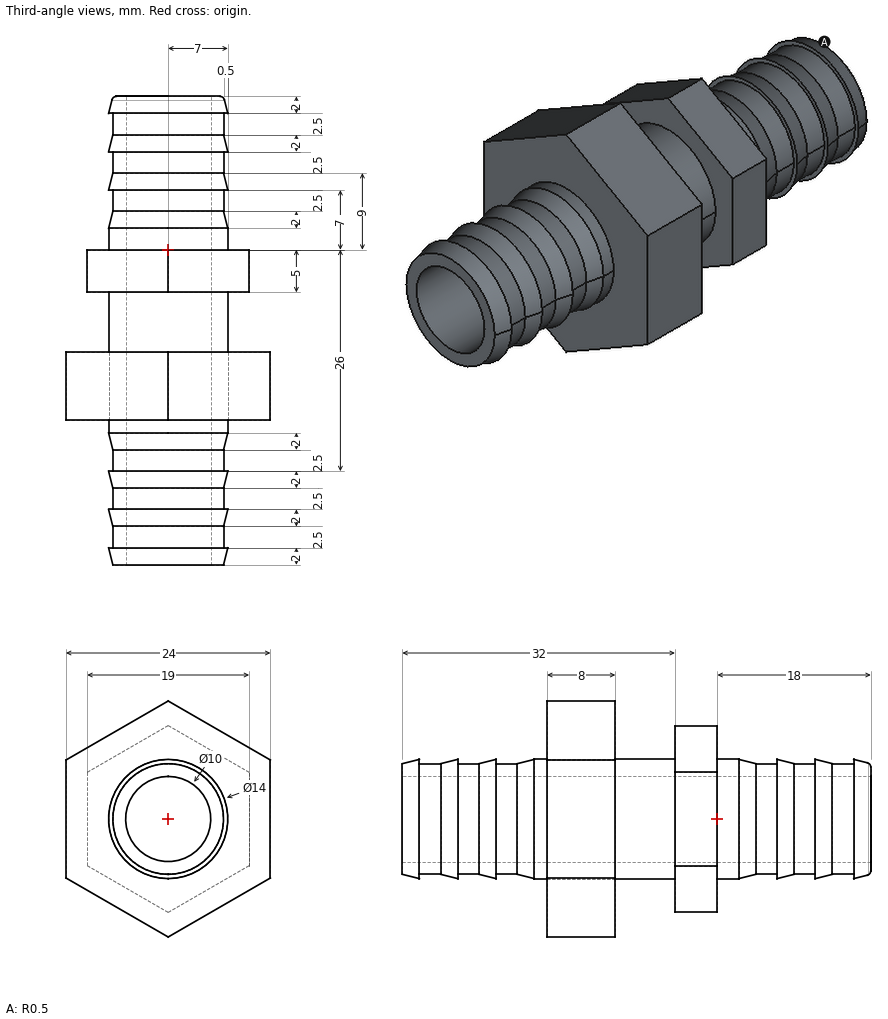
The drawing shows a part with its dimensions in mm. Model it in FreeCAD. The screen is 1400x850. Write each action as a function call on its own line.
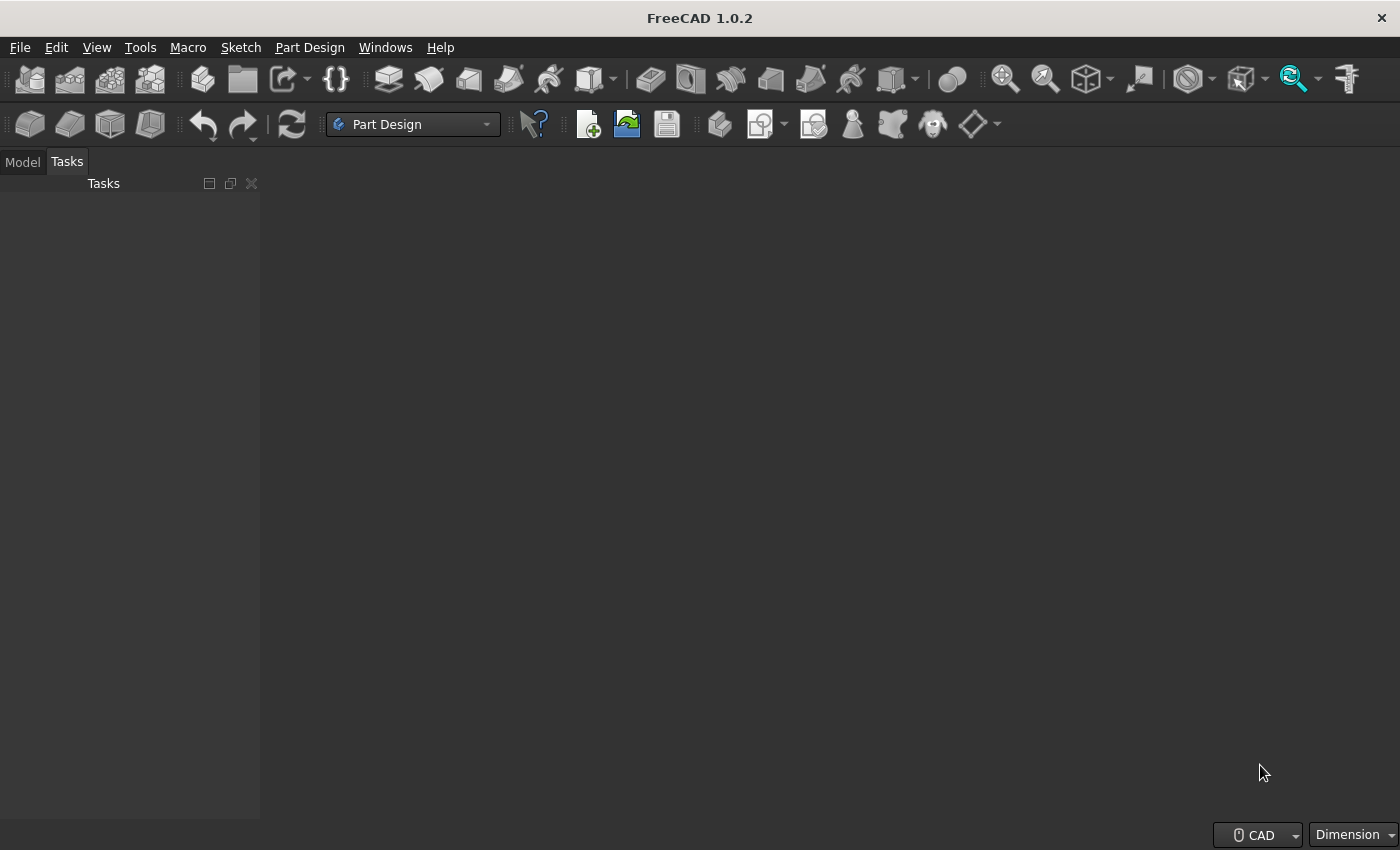
click(588, 124)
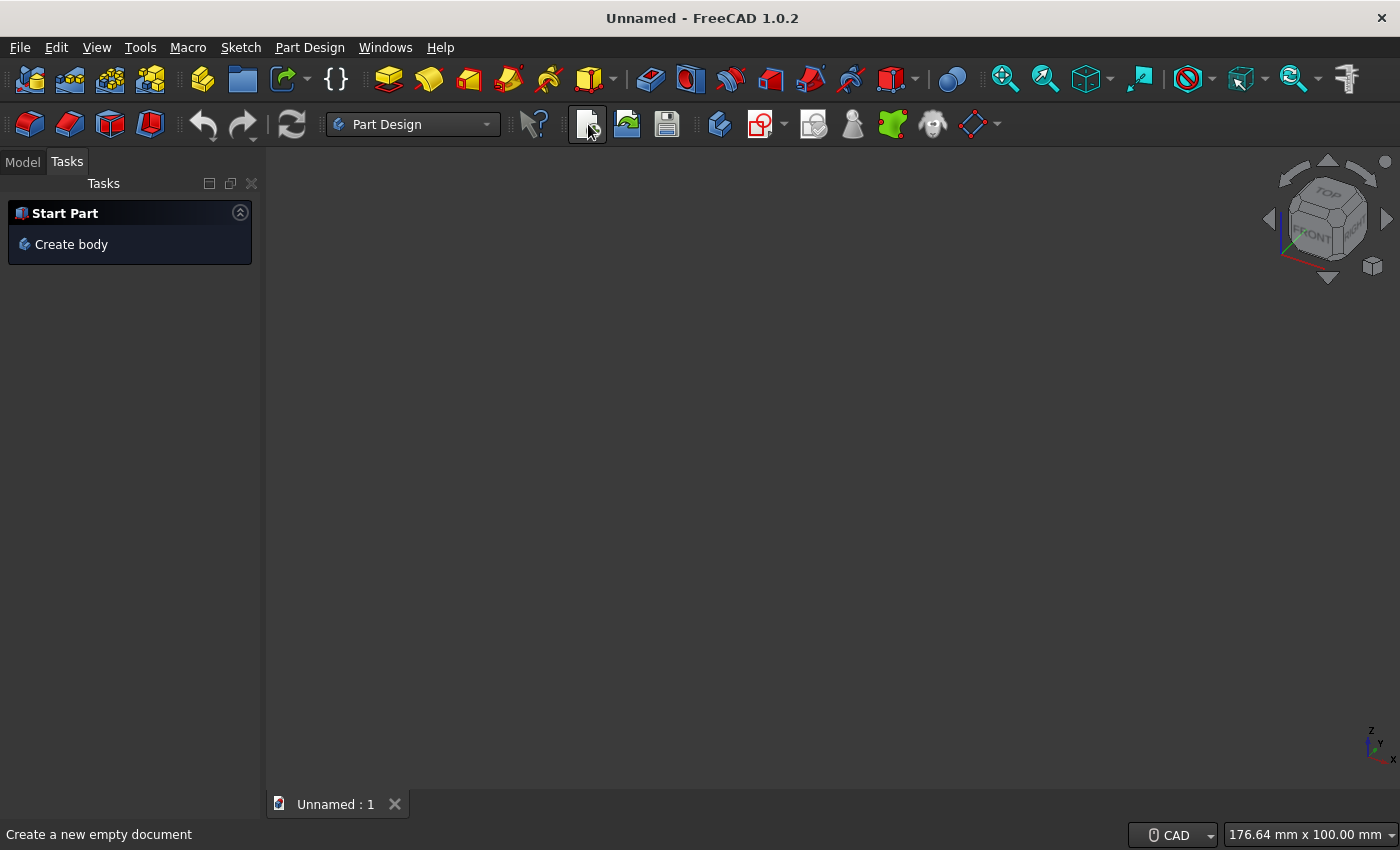
click(760, 124)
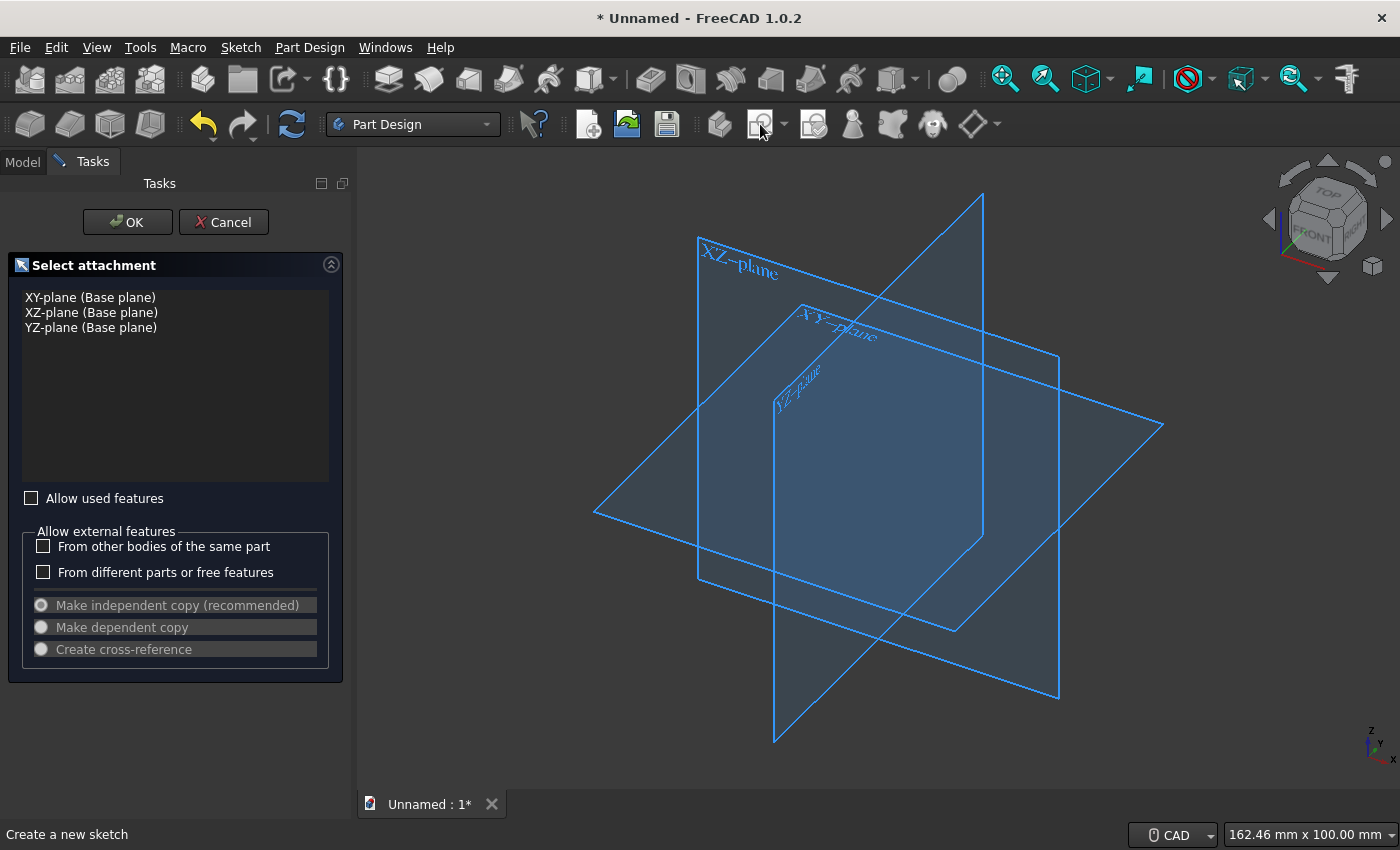
click(82, 312)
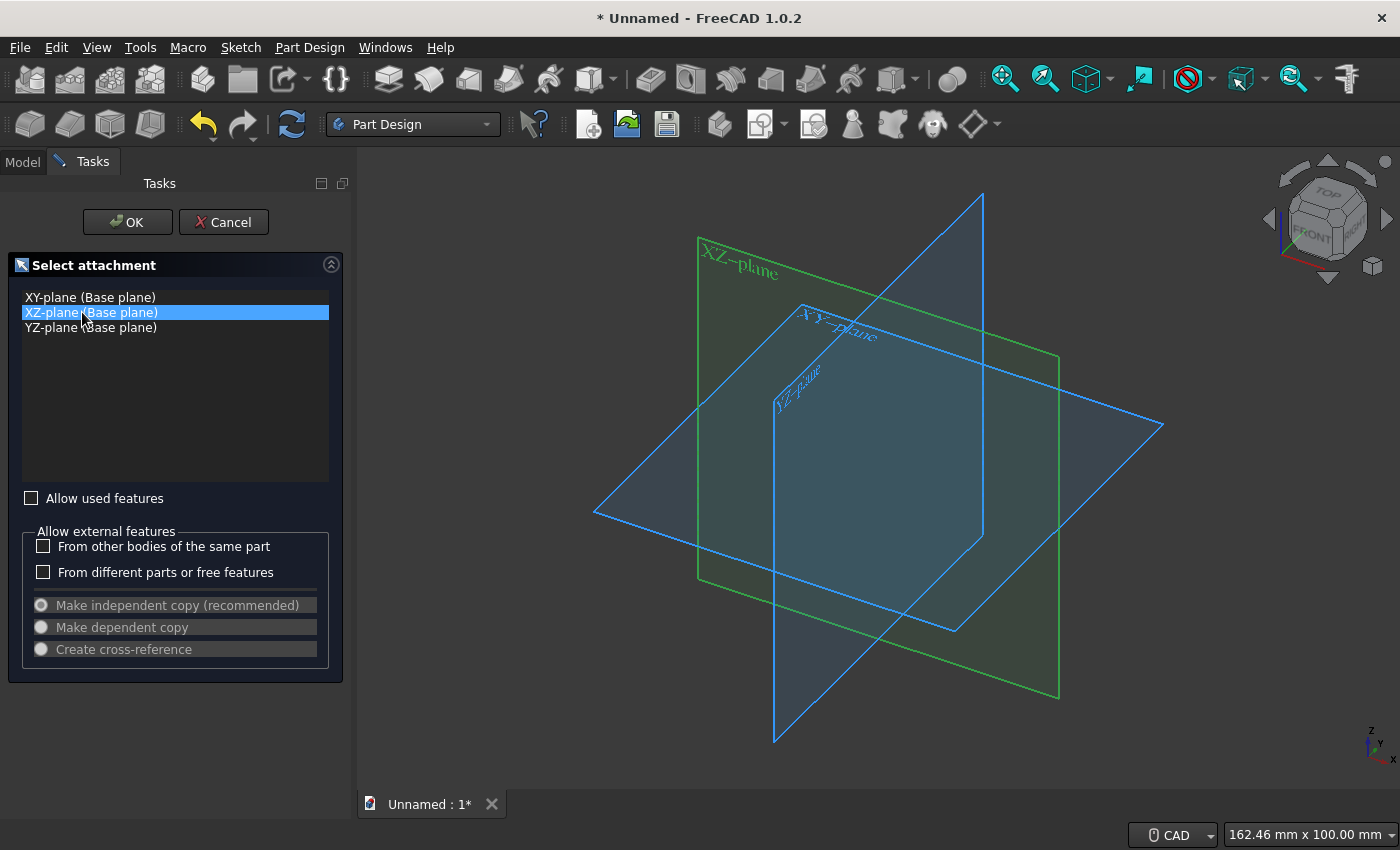
click(128, 222)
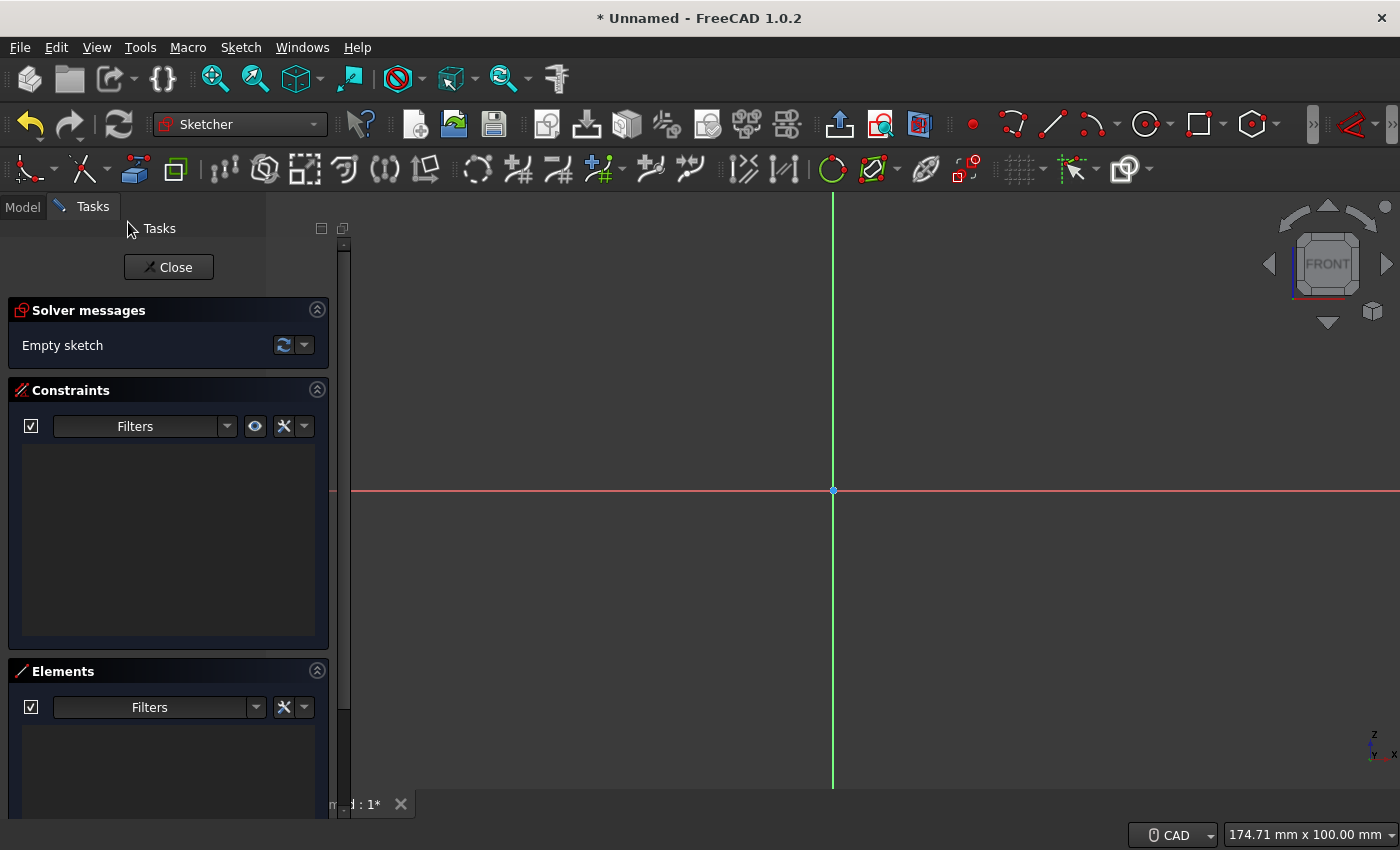
scroll(850, 490, up, 8)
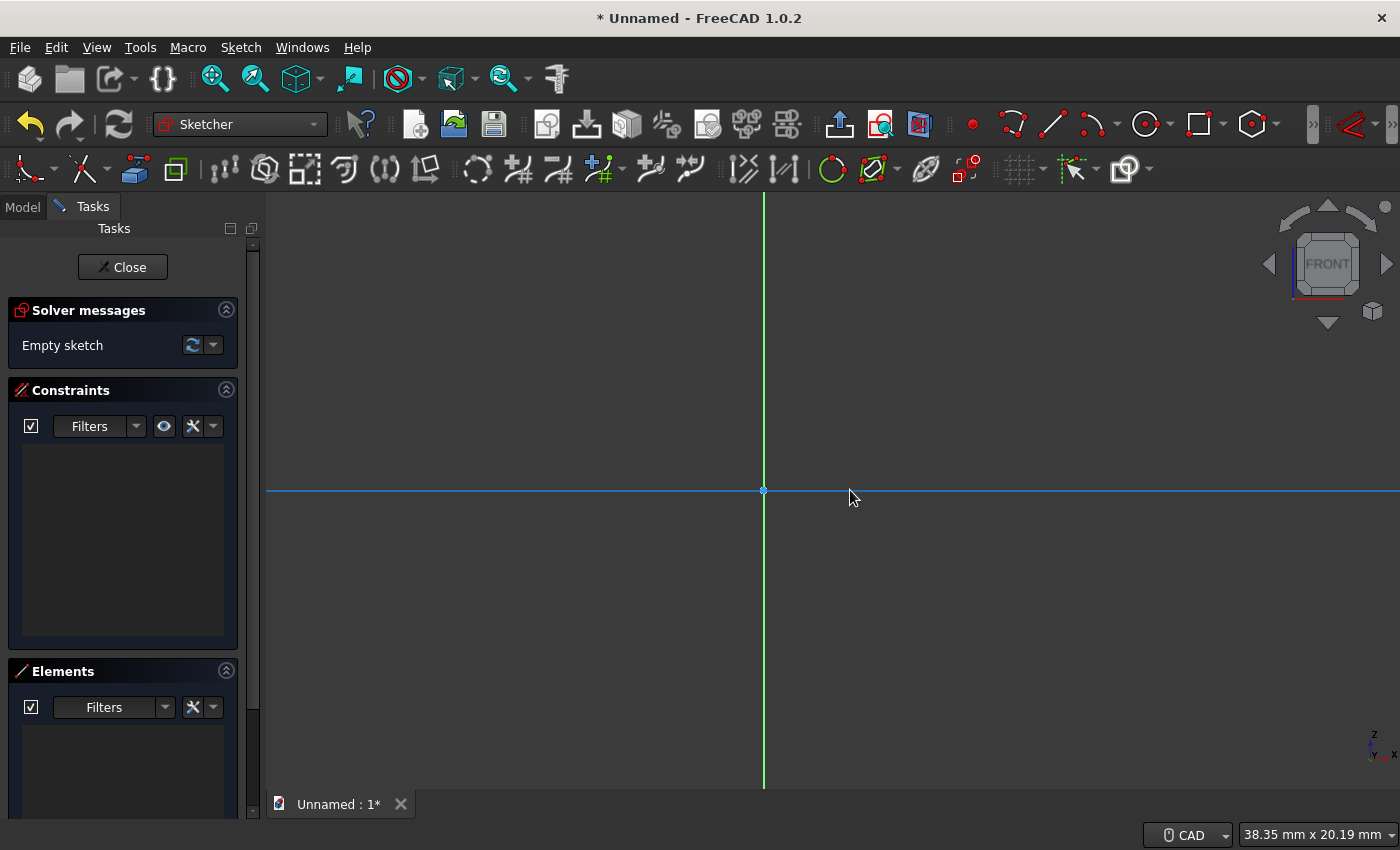
click(1146, 124)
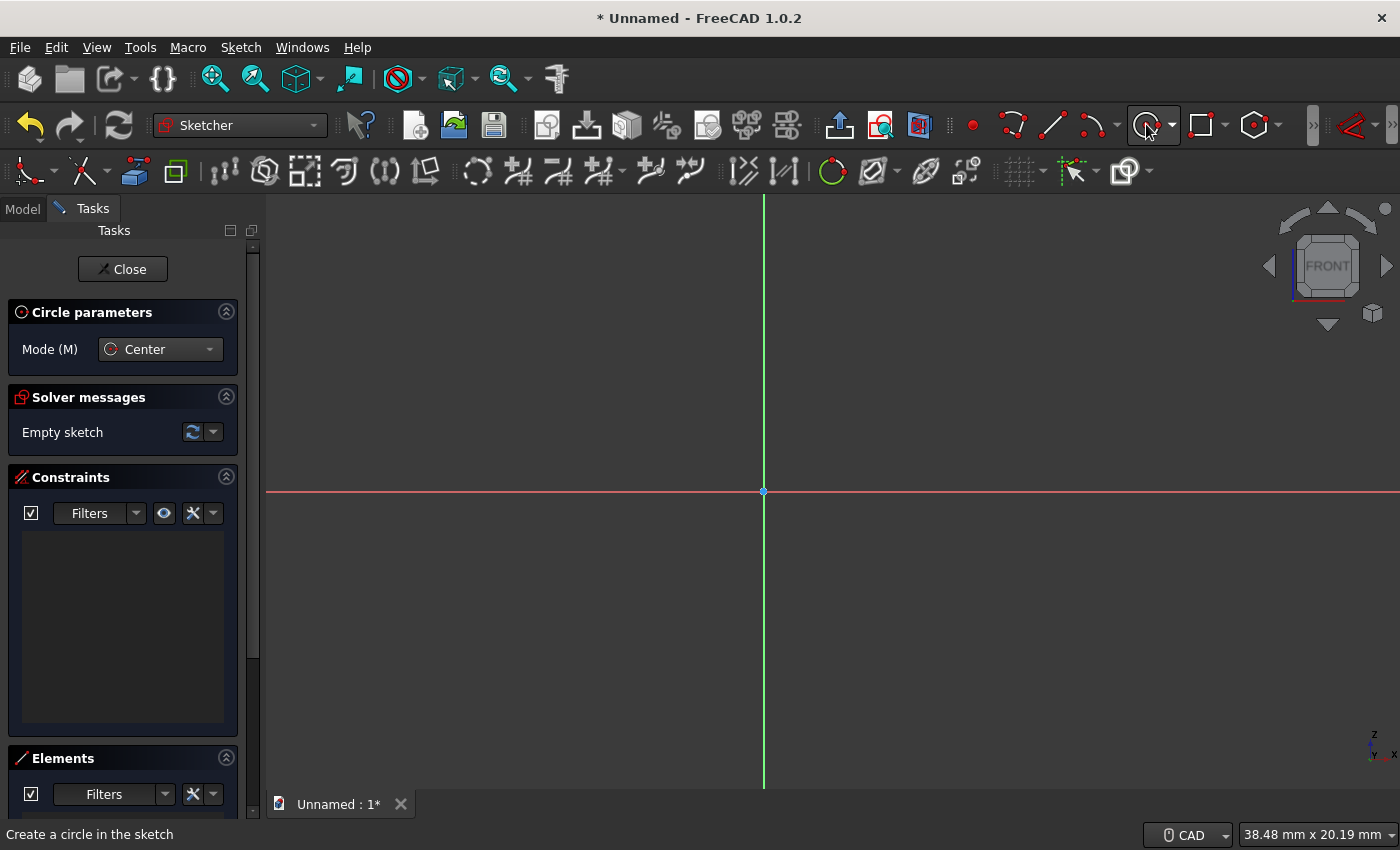
click(764, 492)
move(910, 346)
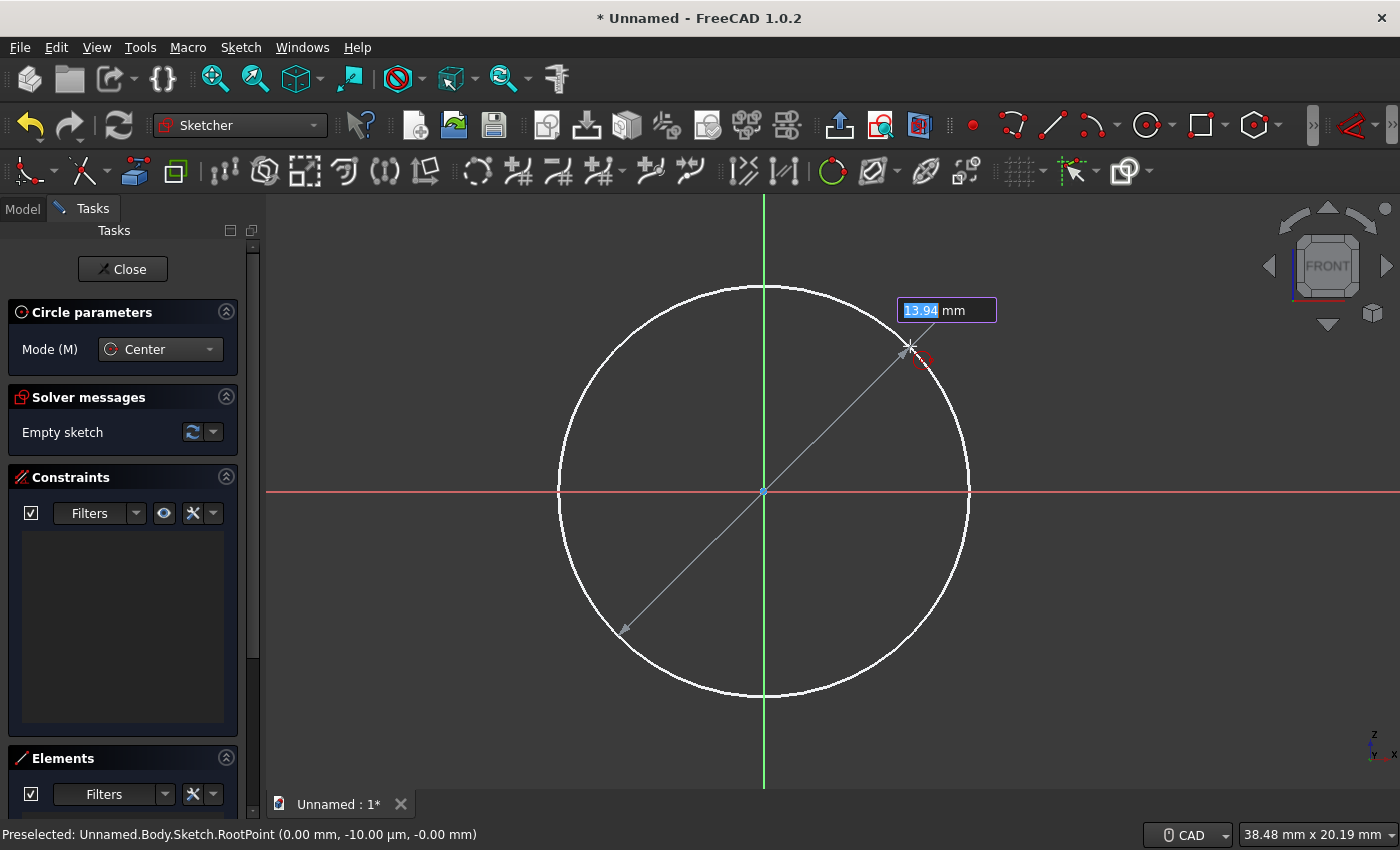
text(14)
key(Return)
key(Escape)